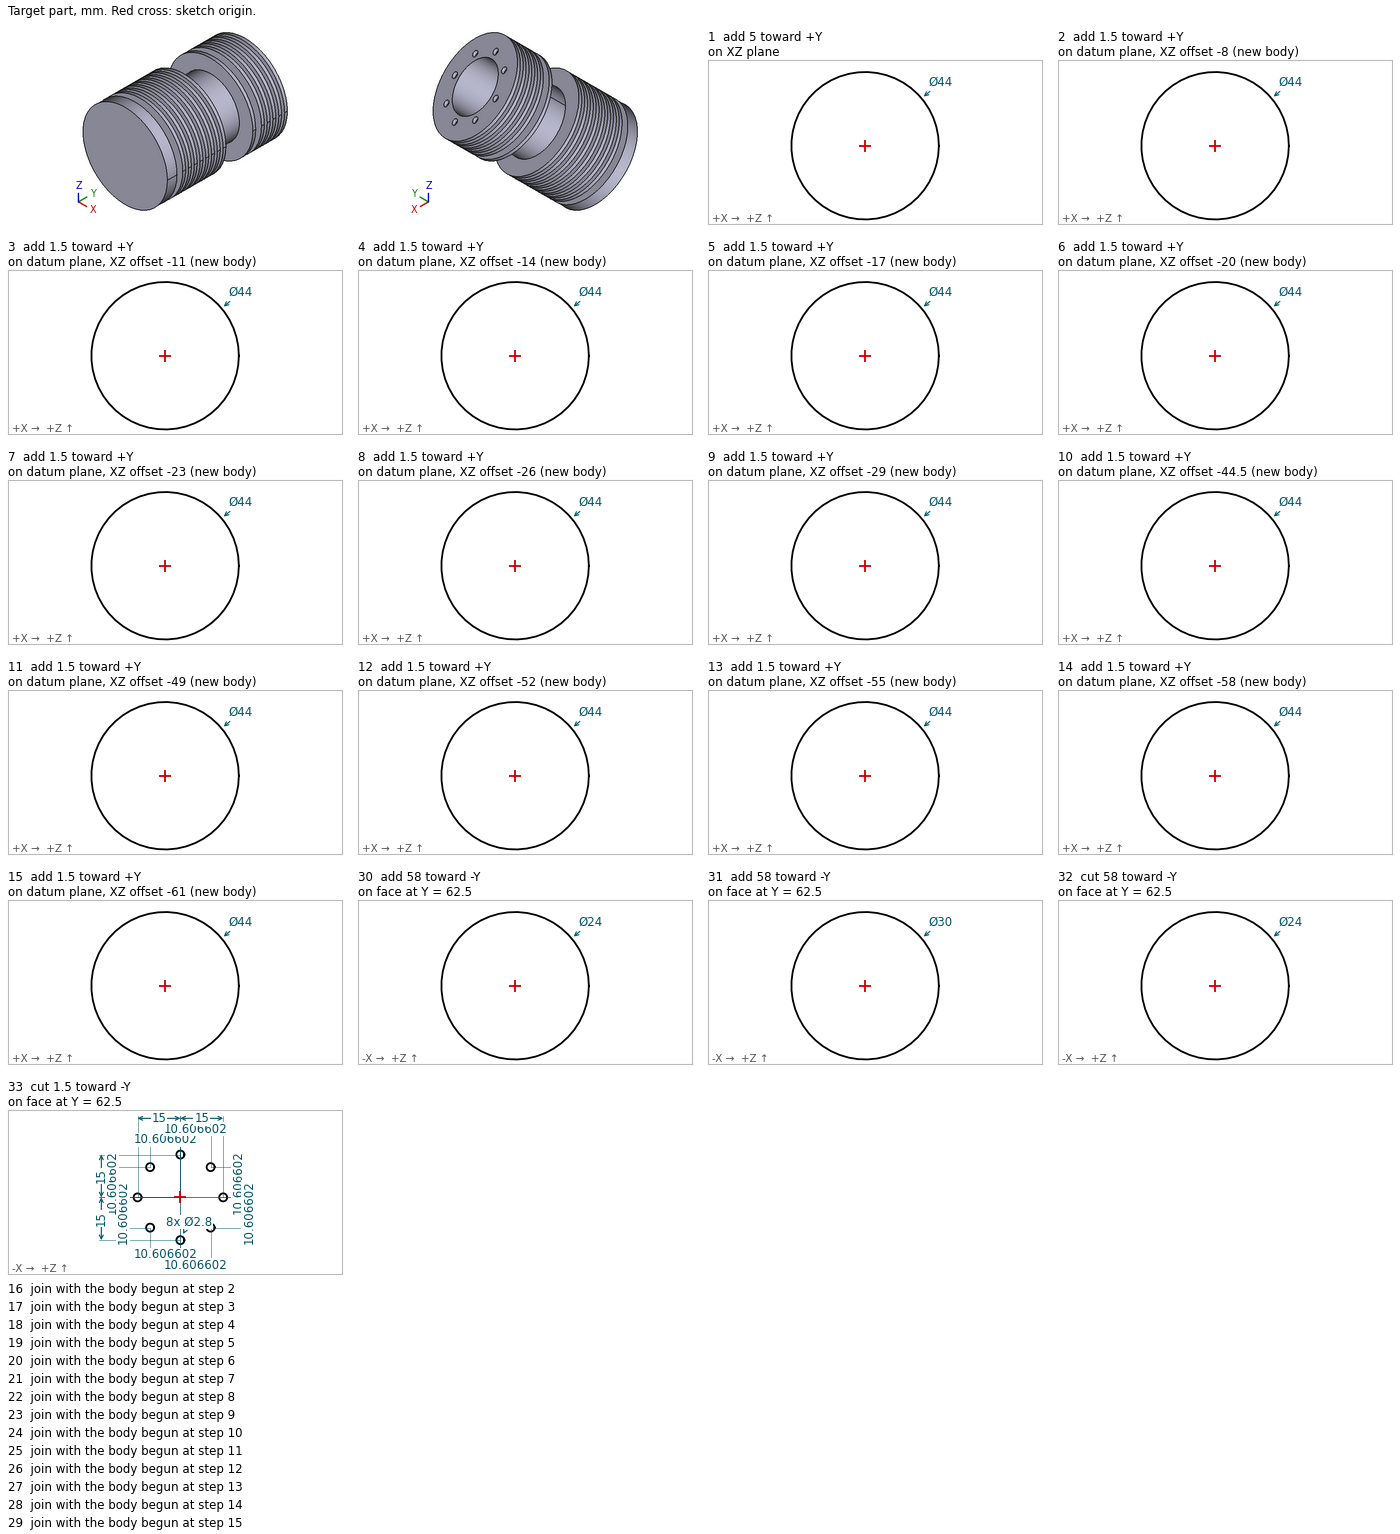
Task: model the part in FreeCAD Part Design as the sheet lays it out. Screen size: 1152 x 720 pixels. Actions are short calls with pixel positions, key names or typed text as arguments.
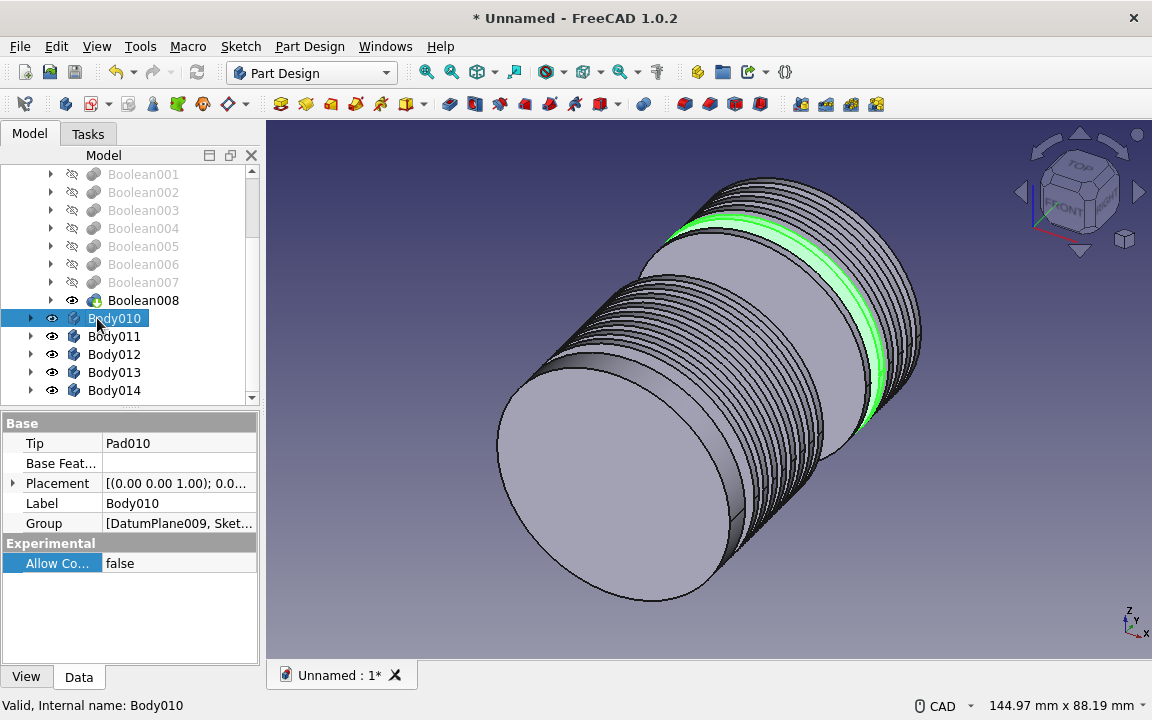
click(644, 104)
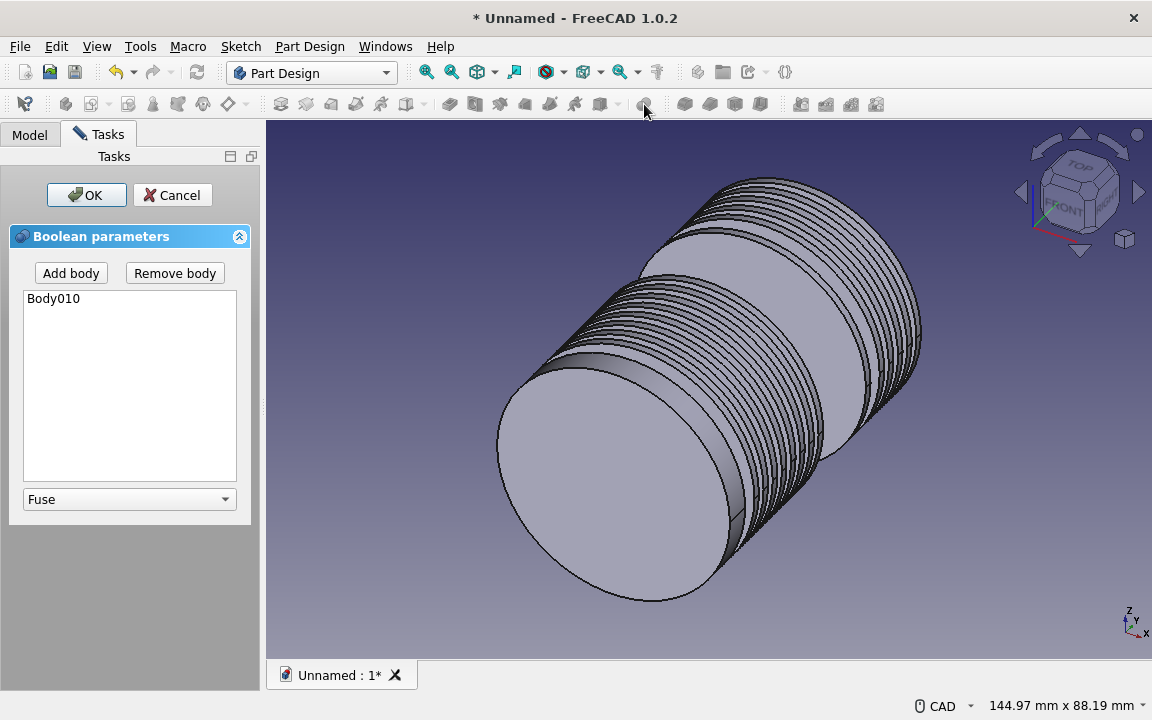
click(87, 195)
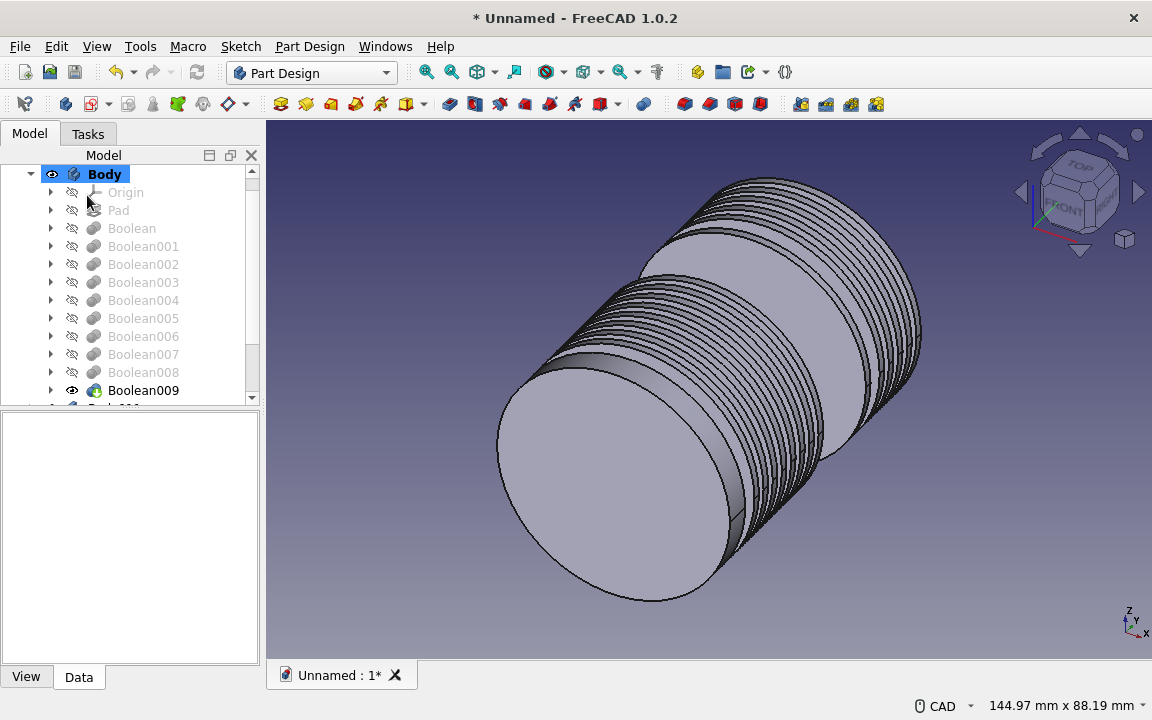
scroll(121, 278, down, 3)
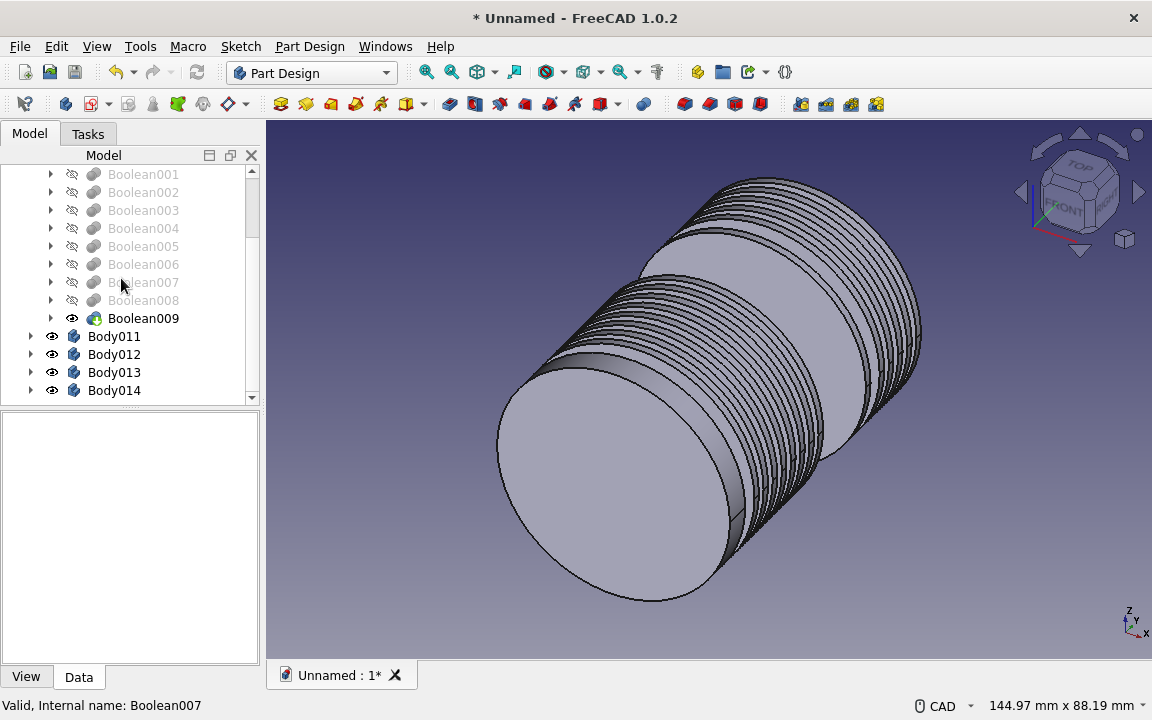
click(97, 336)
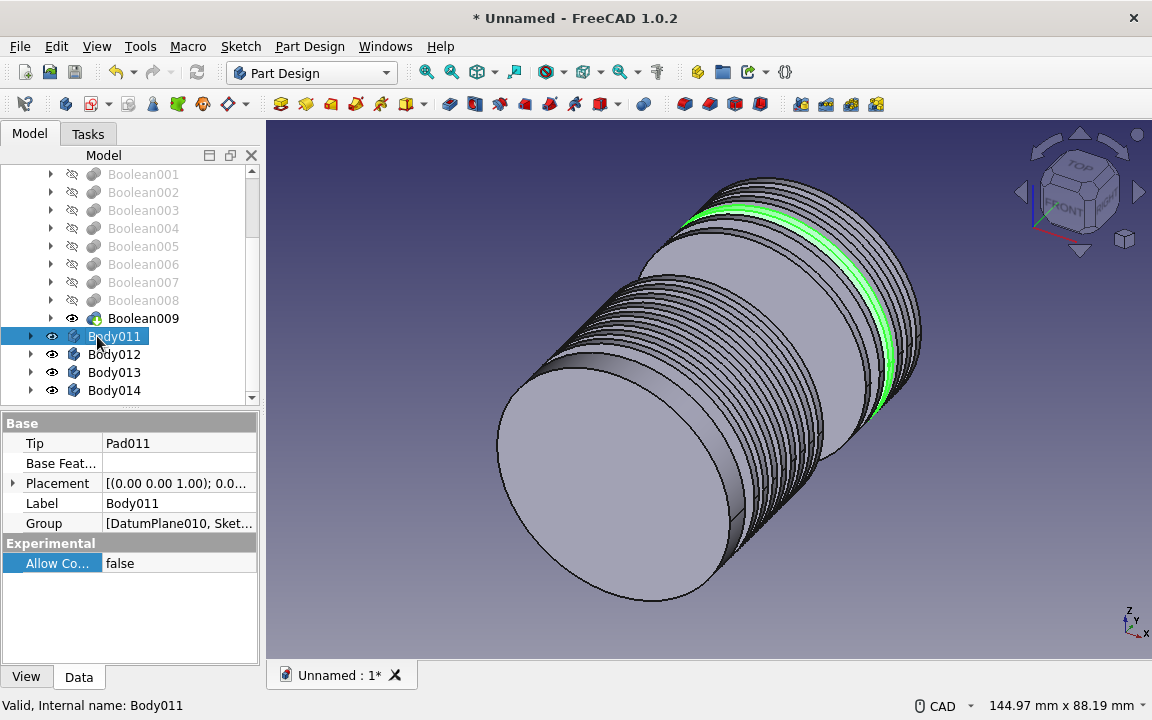
click(644, 104)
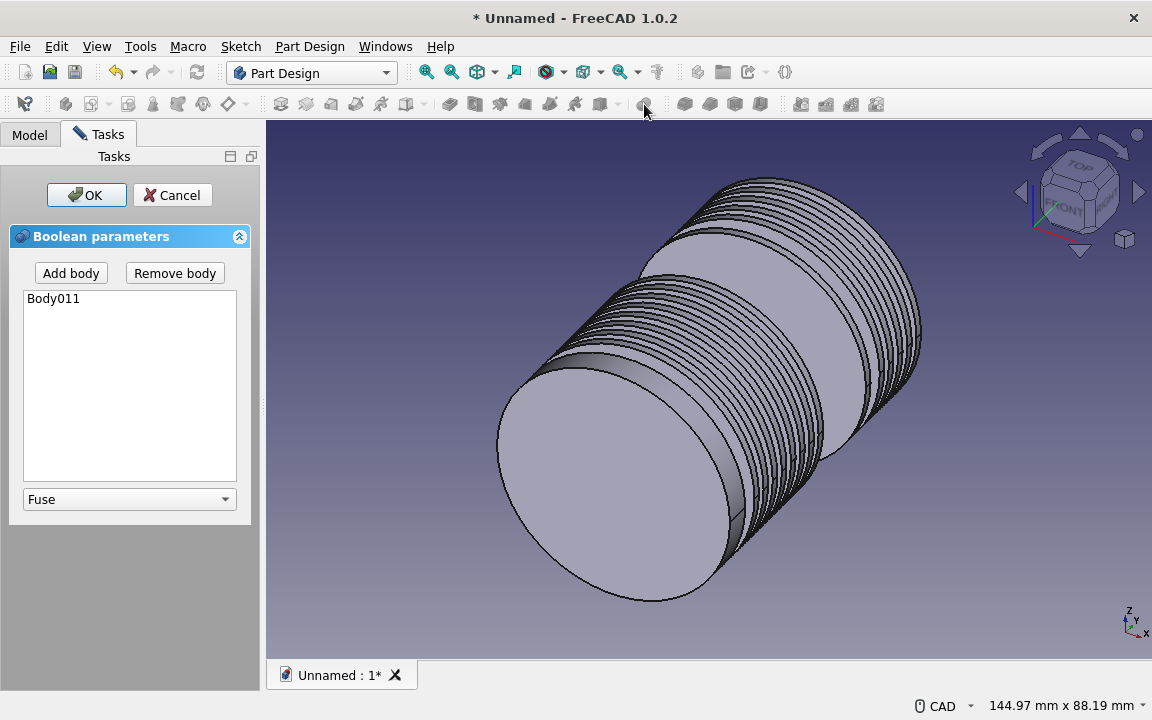
click(87, 195)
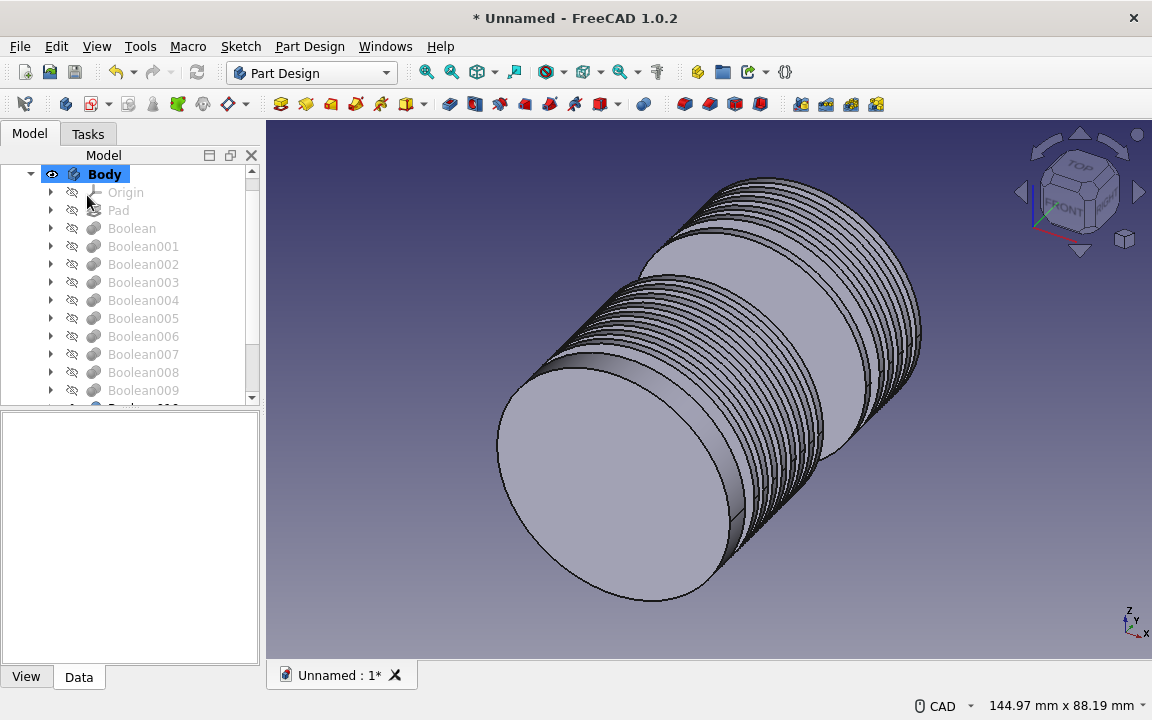
scroll(121, 278, down, 3)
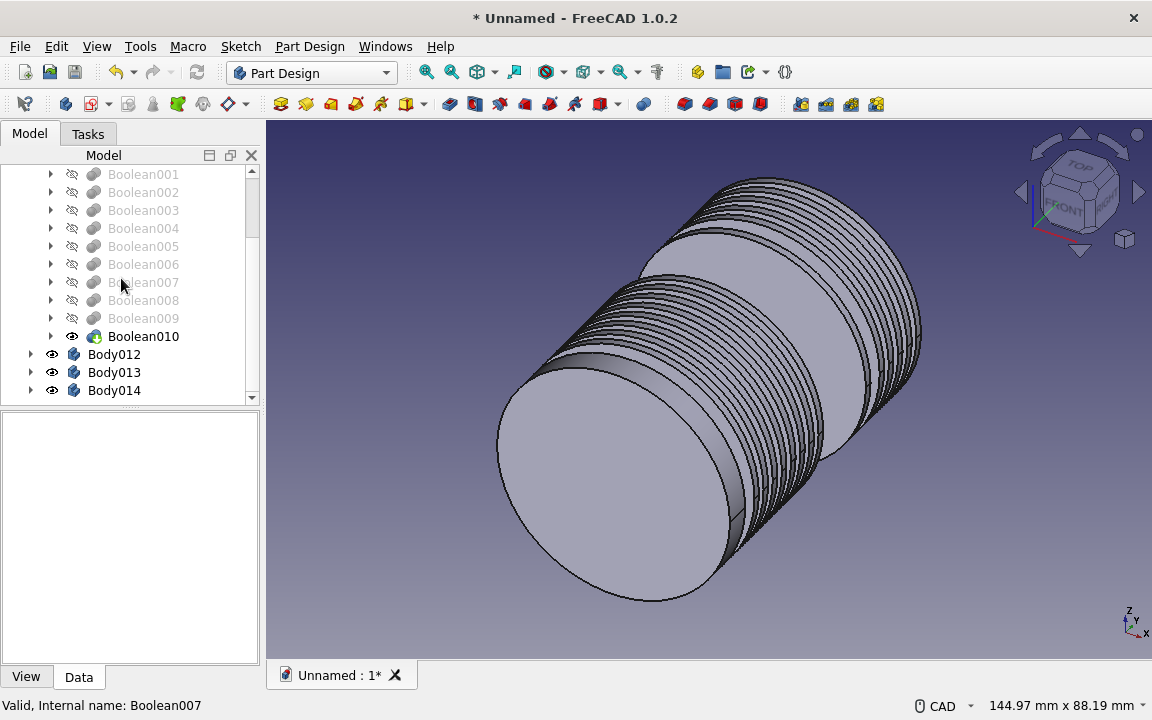
click(97, 354)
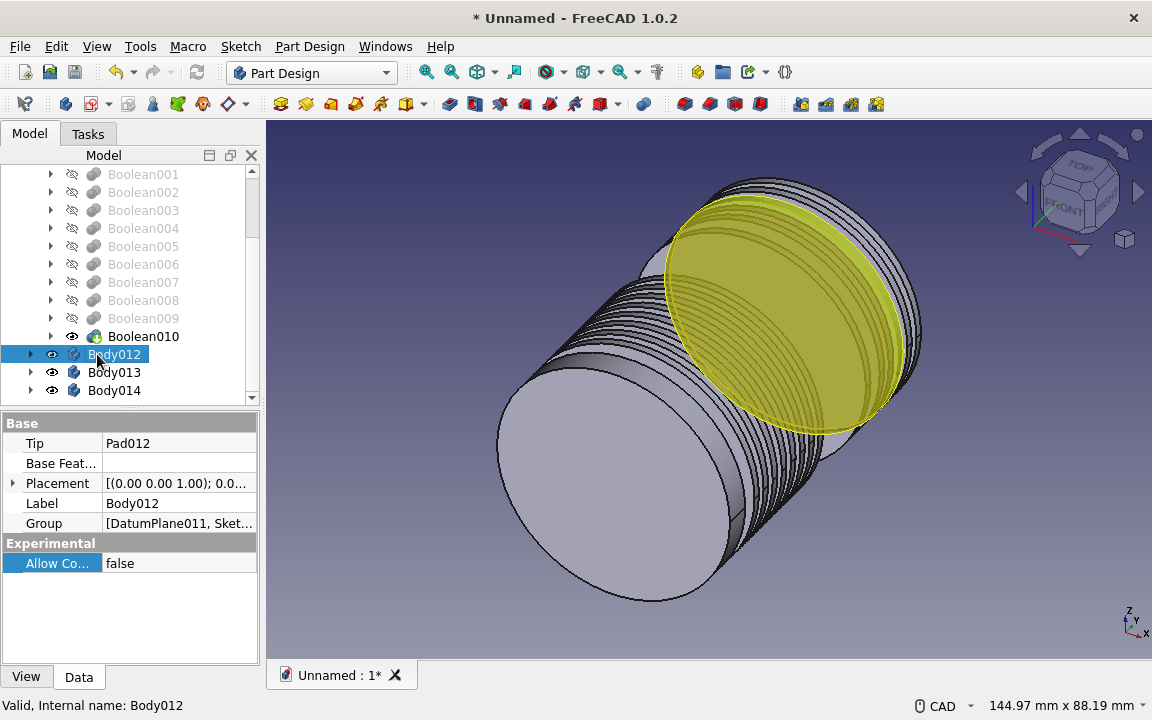
click(644, 104)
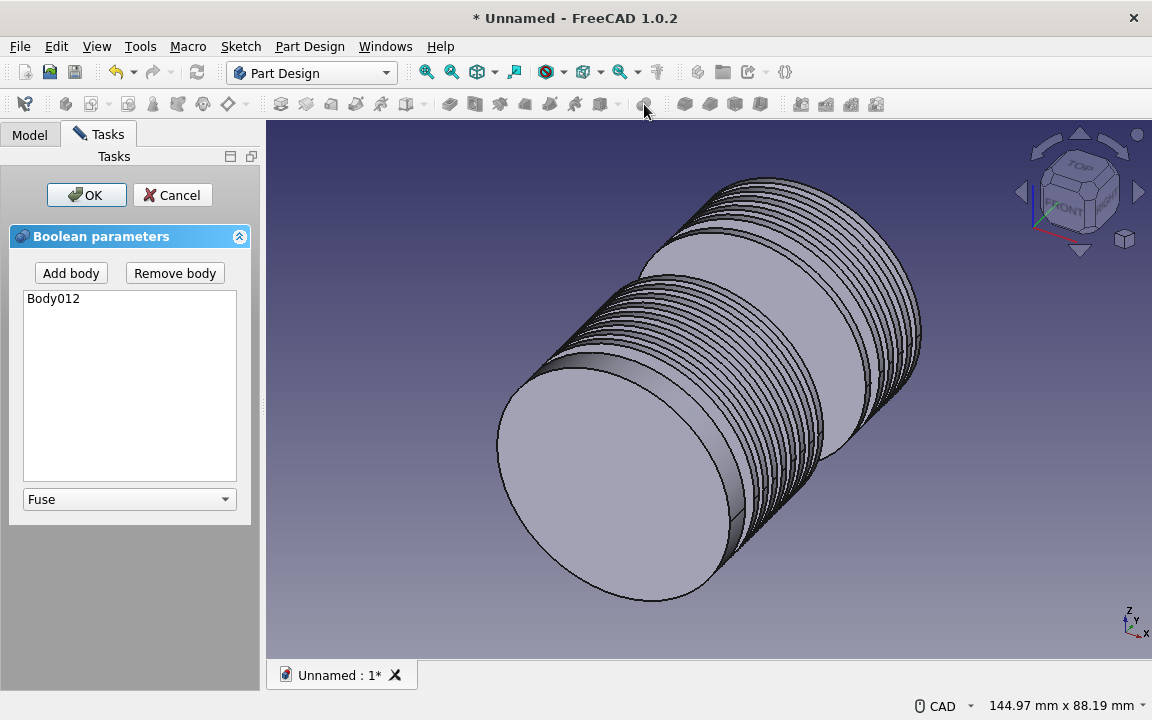
click(87, 195)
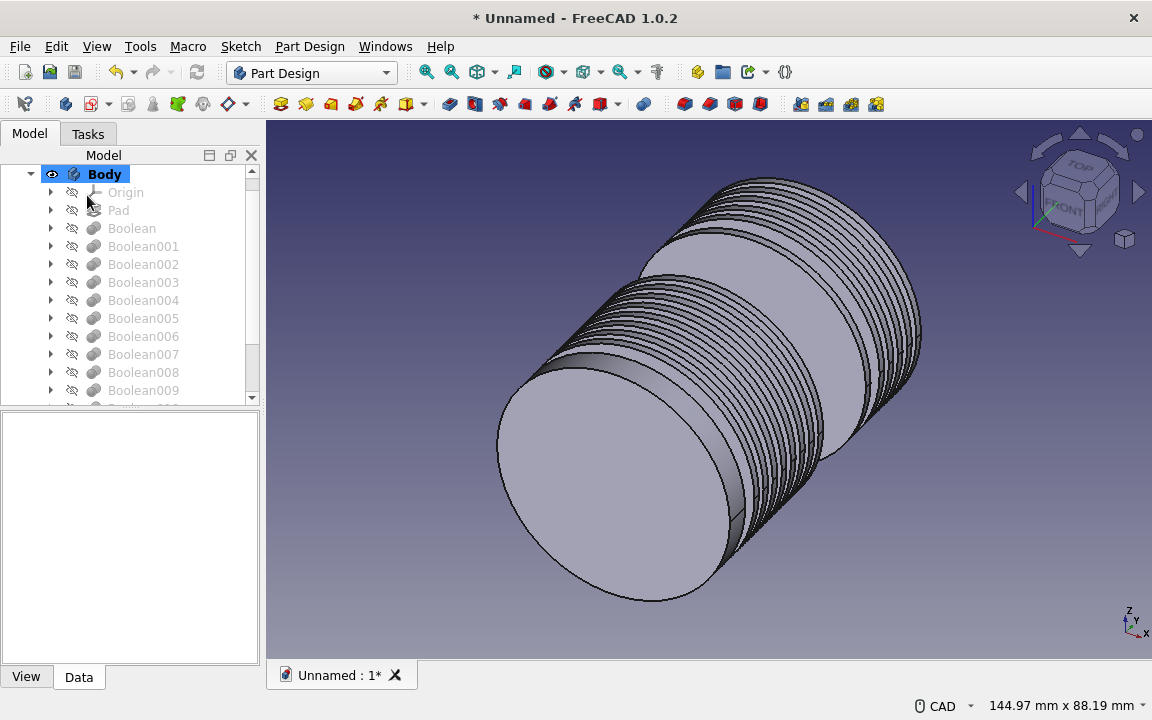
scroll(121, 278, down, 3)